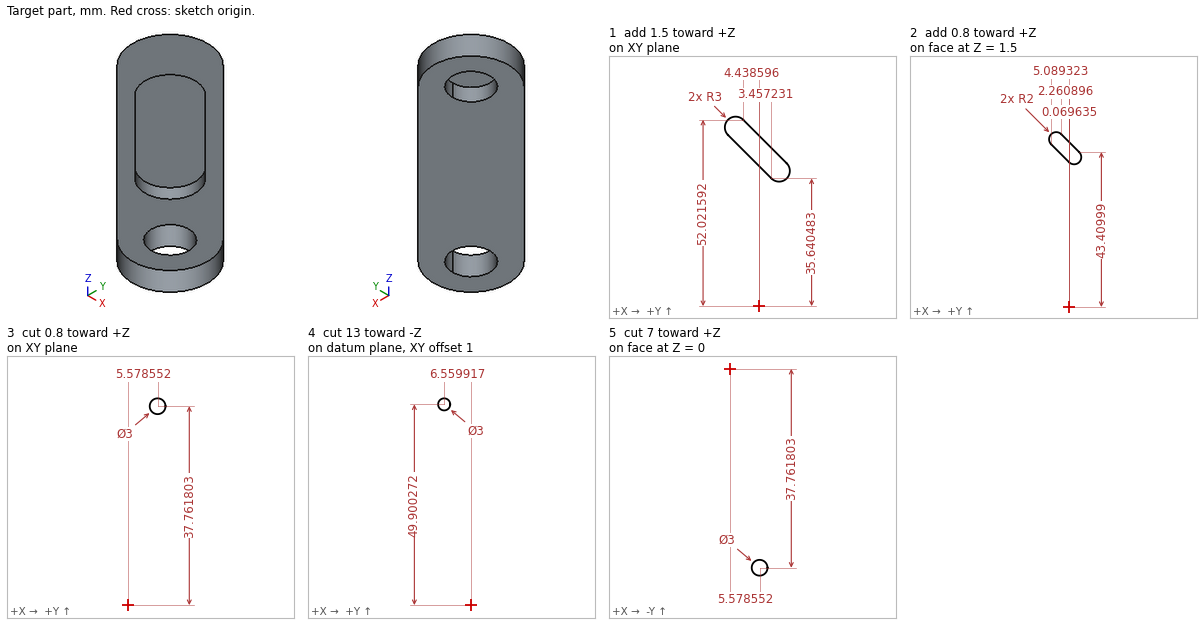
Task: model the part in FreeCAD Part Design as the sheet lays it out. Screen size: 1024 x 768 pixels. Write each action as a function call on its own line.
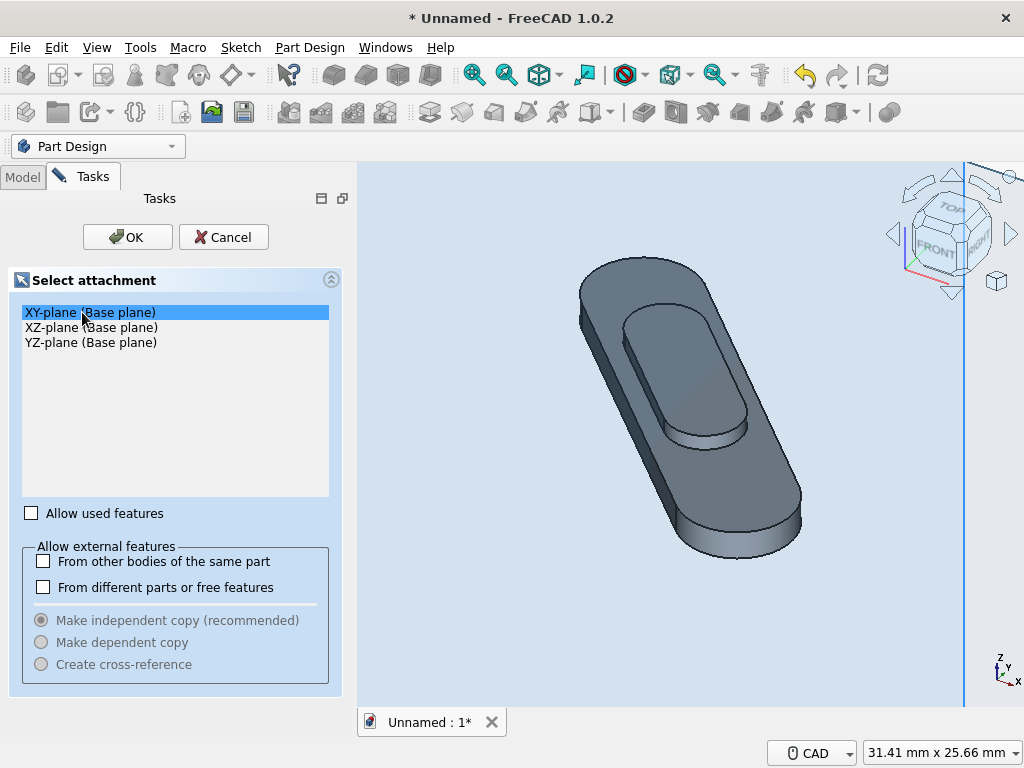
click(128, 237)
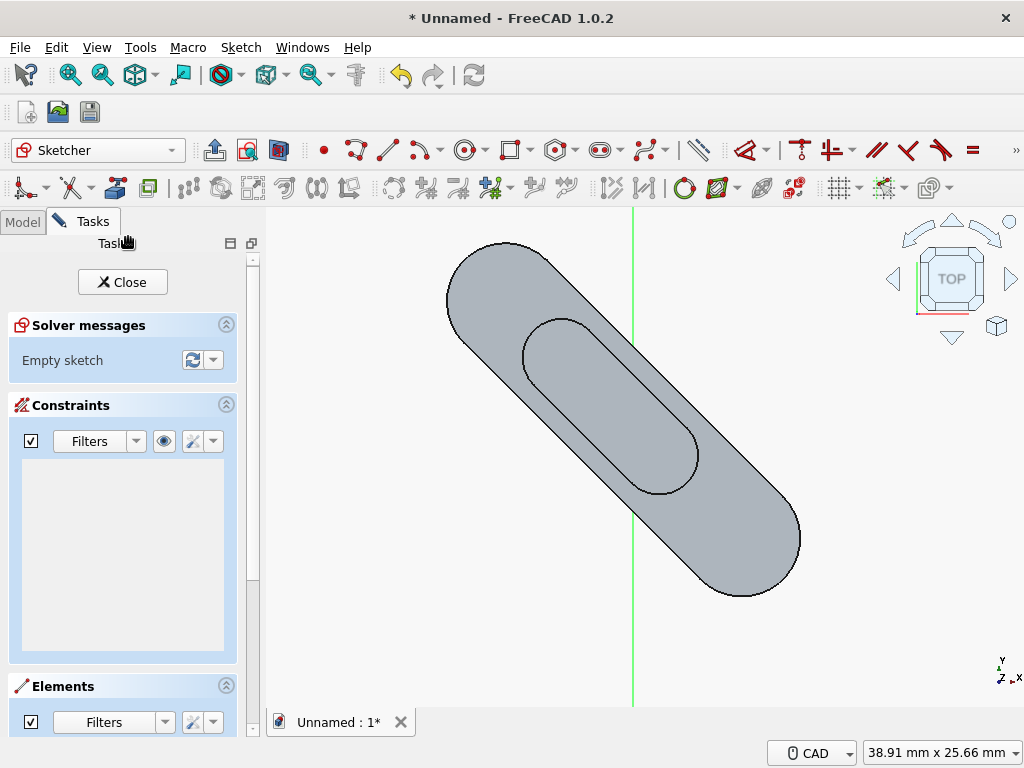
click(280, 150)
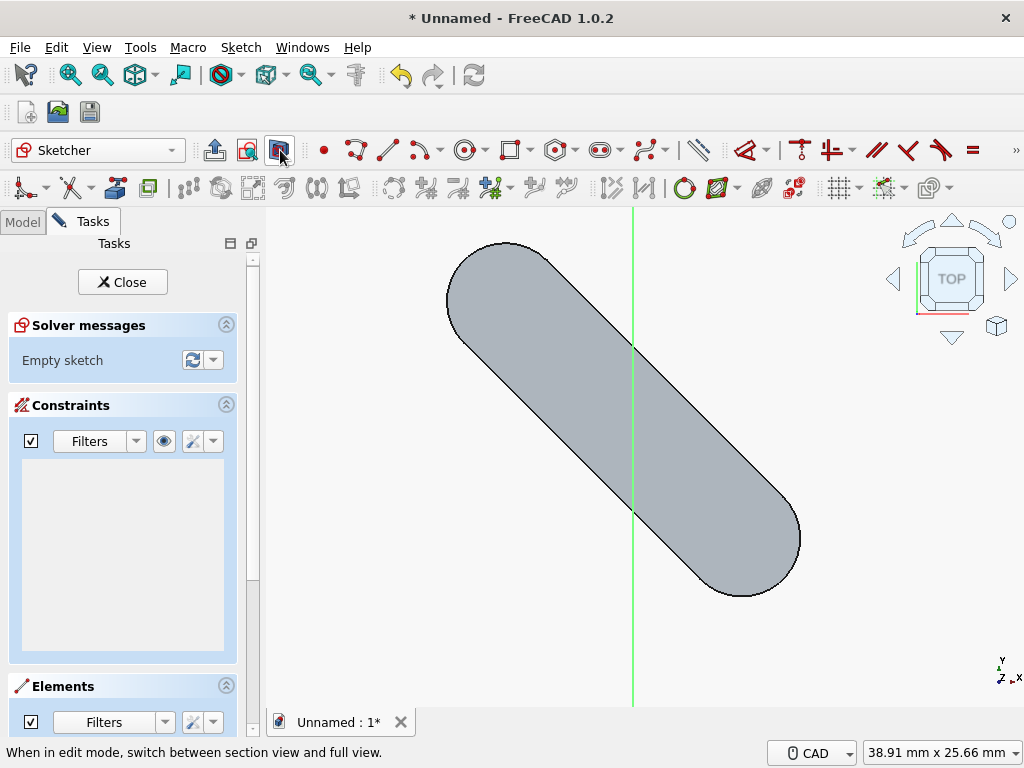
scroll(784, 559, up, 8)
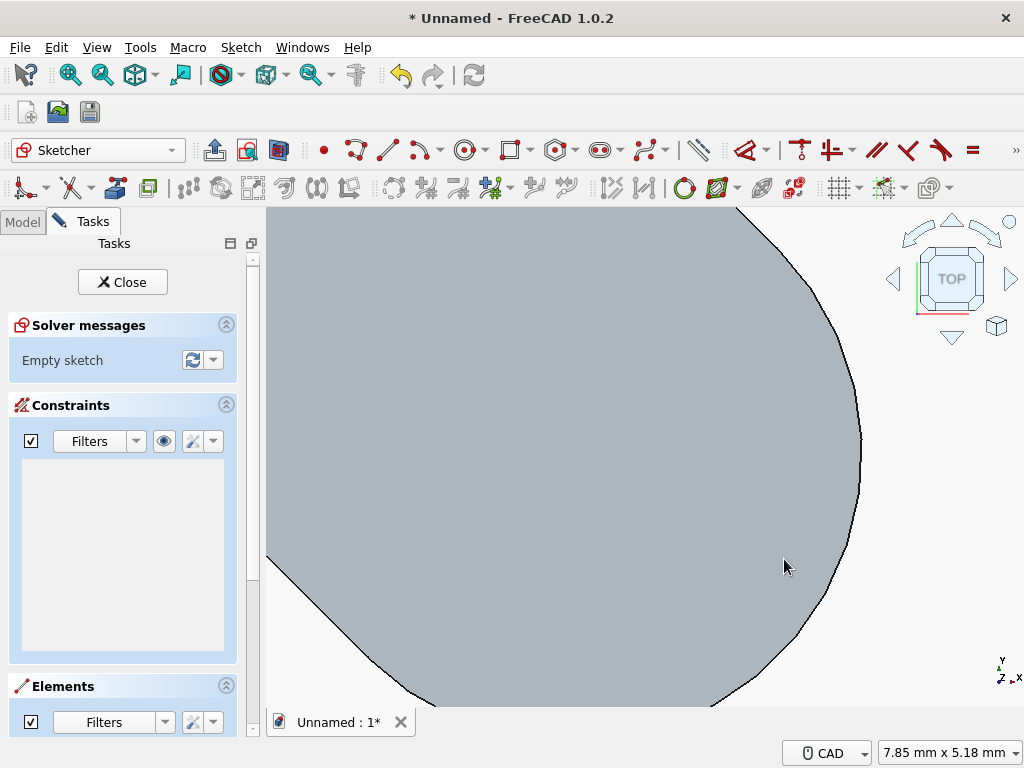
click(466, 150)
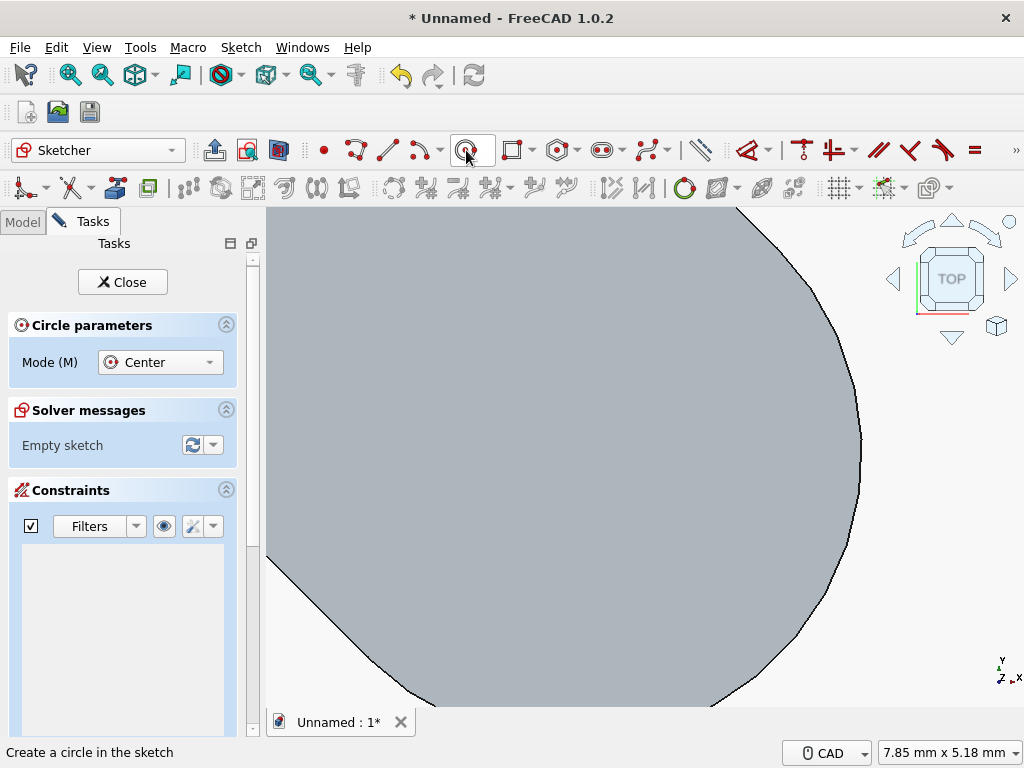
click(572, 453)
click(675, 350)
key(Escape)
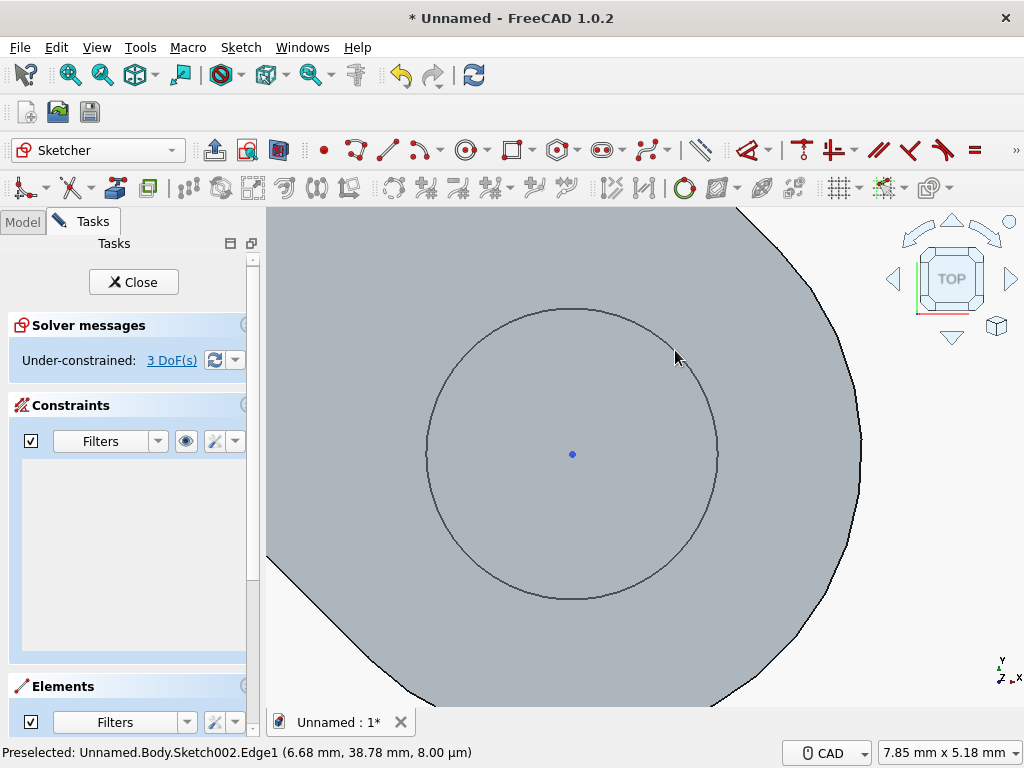
click(748, 150)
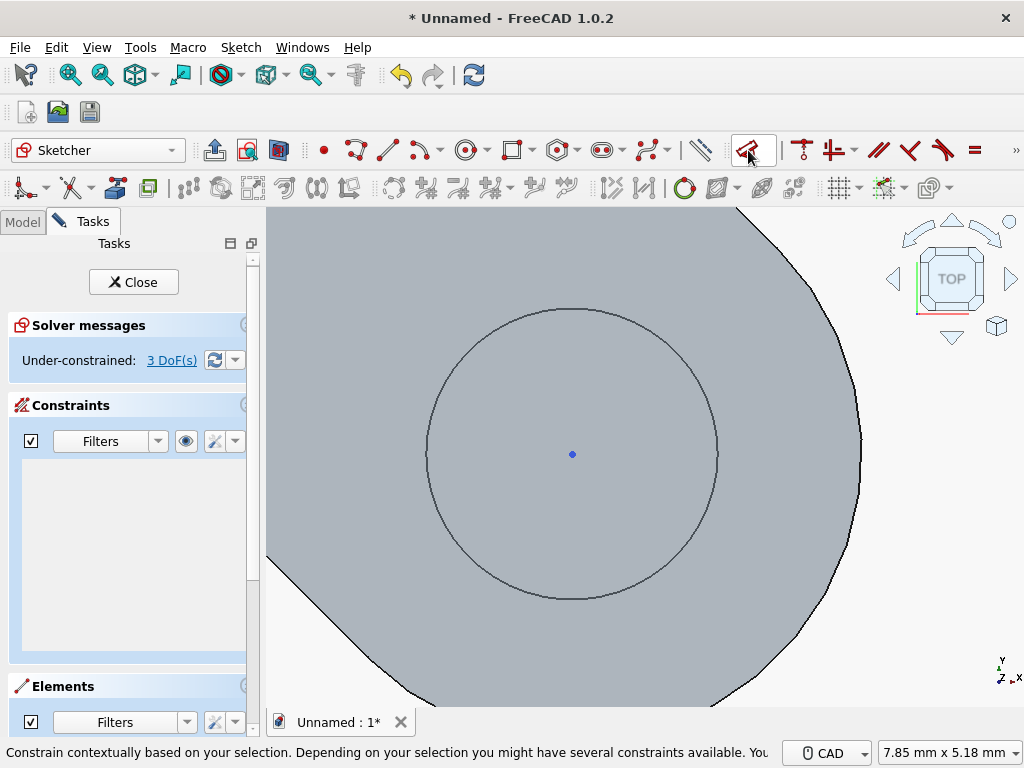
click(675, 351)
click(698, 328)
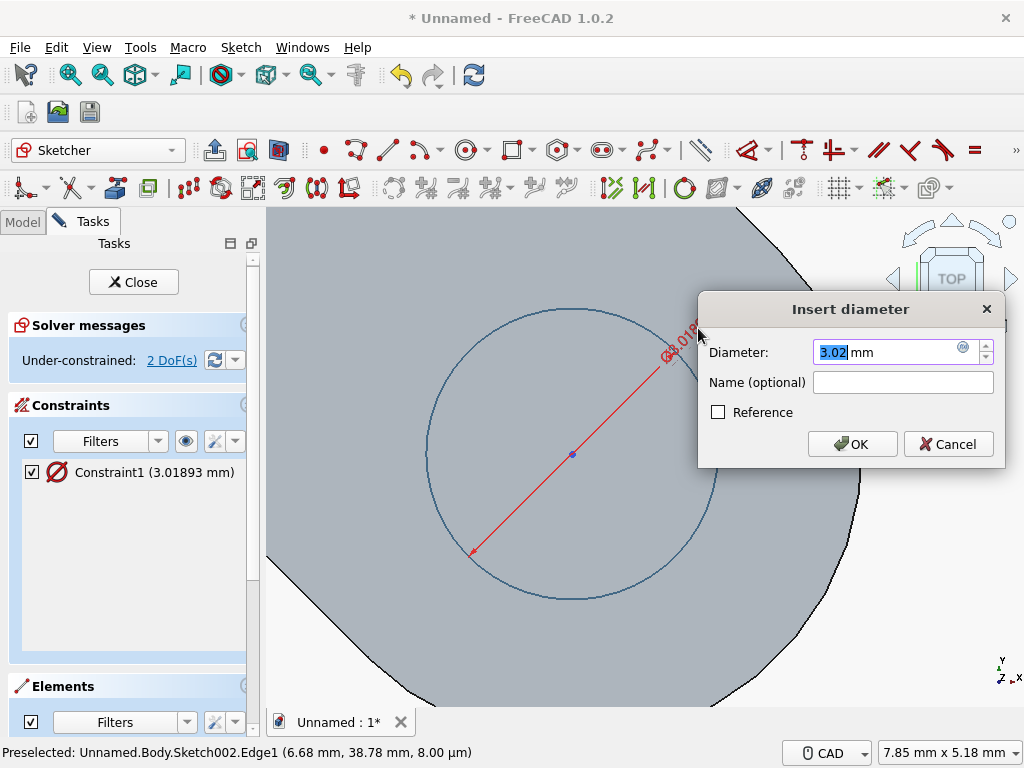
text(3)
key(Return)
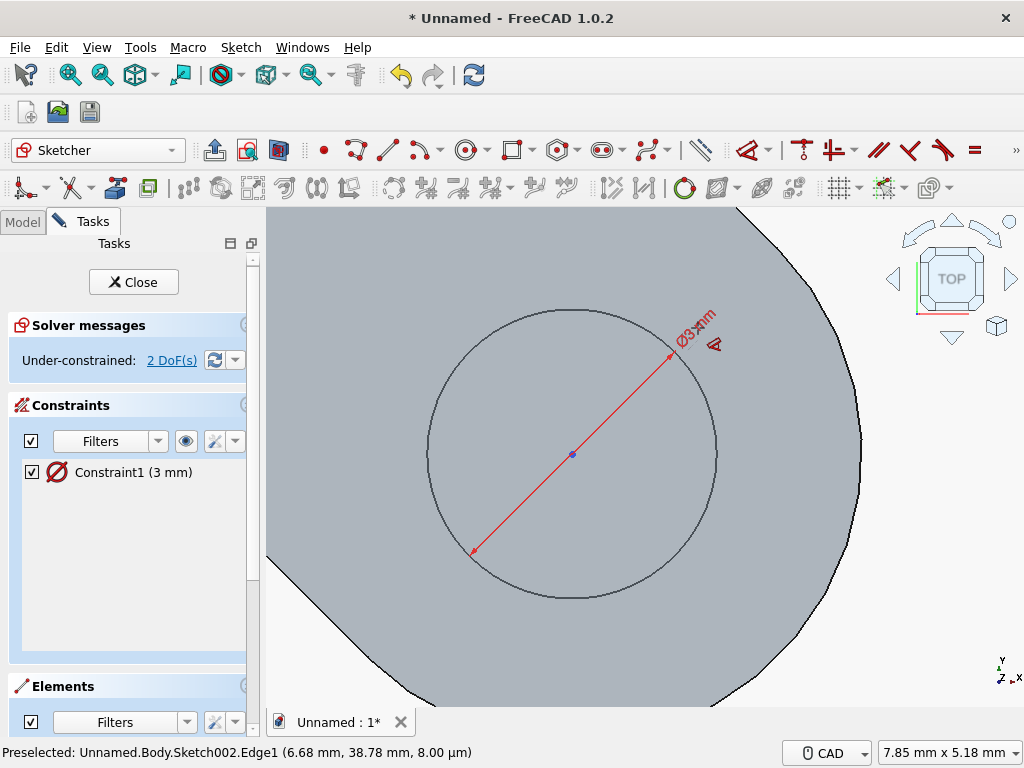
click(572, 454)
click(369, 420)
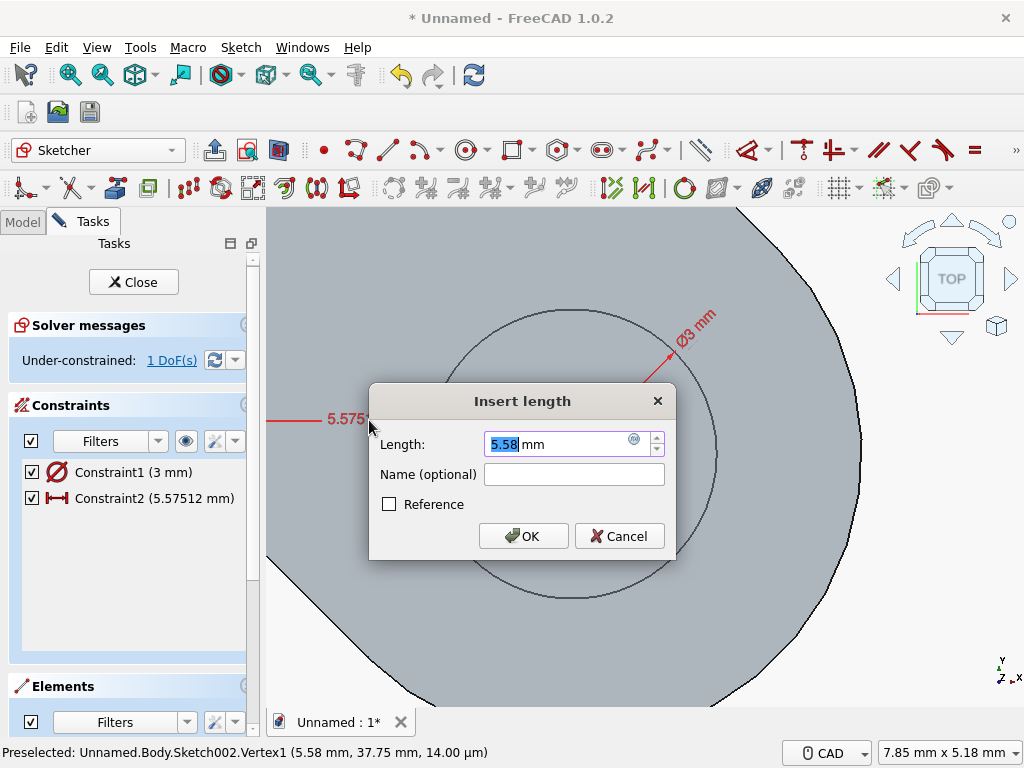
text(5.578552)
key(Return)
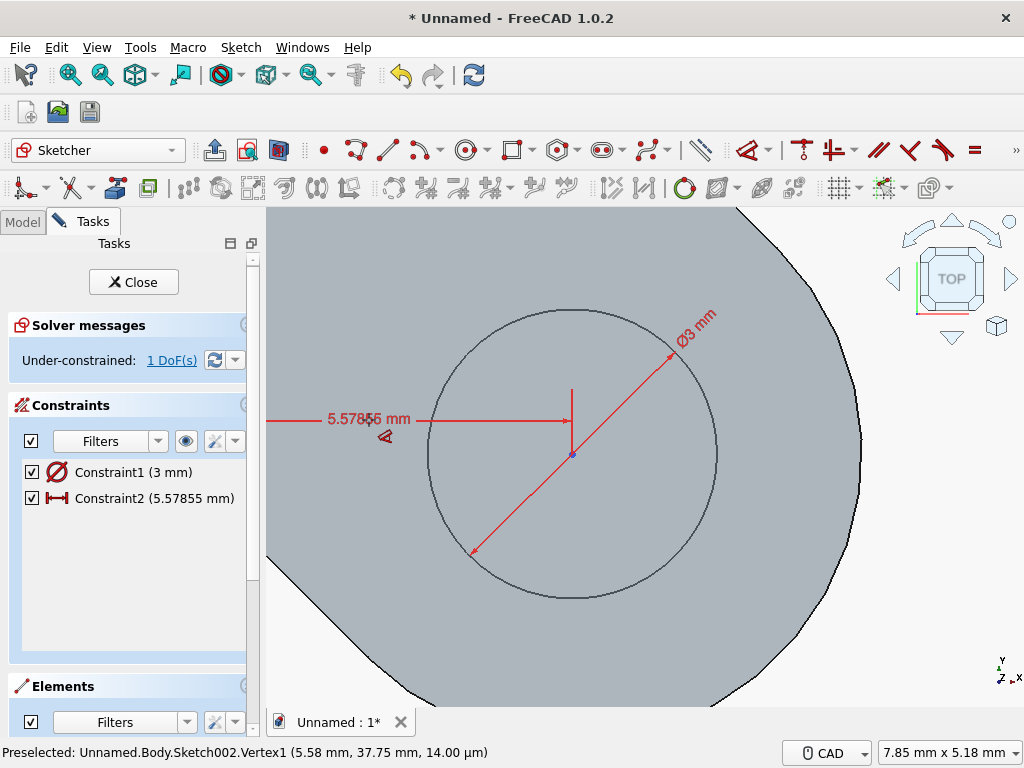
click(572, 454)
click(606, 567)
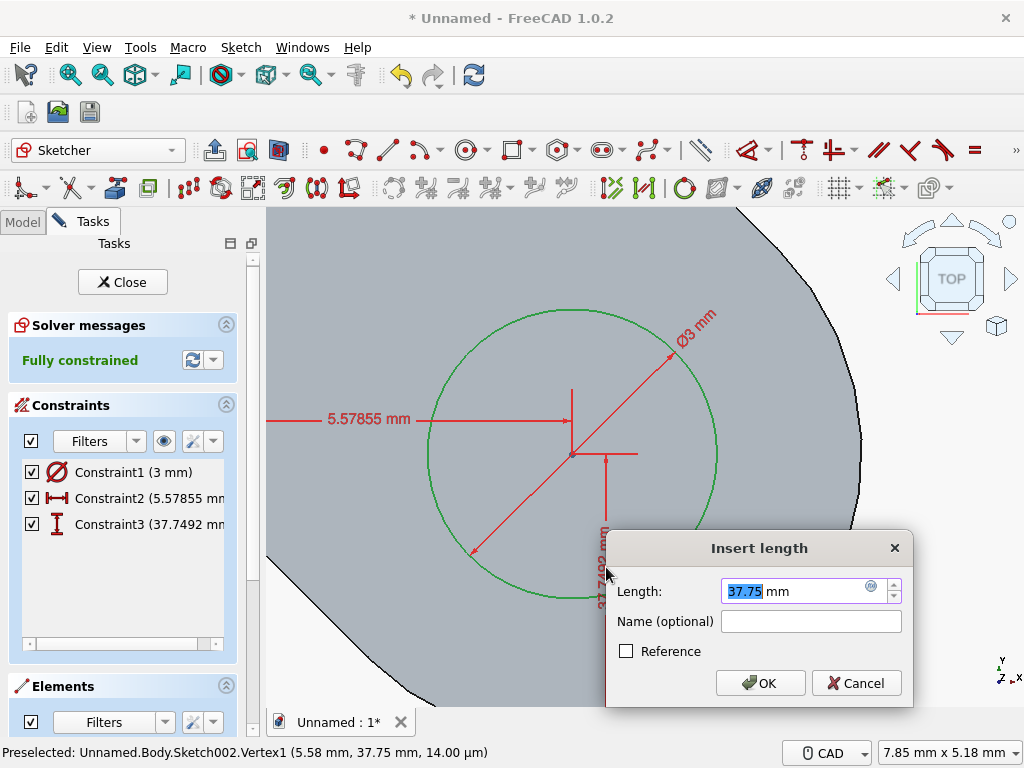
text(37.761803)
key(Return)
key(Escape)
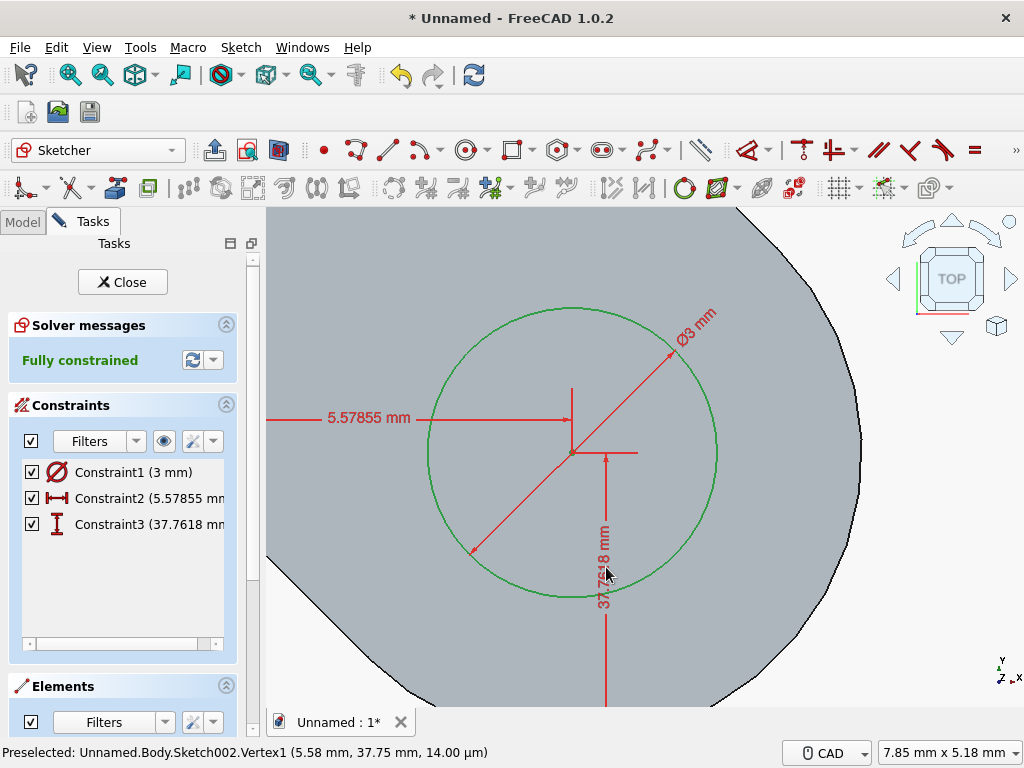
click(123, 282)